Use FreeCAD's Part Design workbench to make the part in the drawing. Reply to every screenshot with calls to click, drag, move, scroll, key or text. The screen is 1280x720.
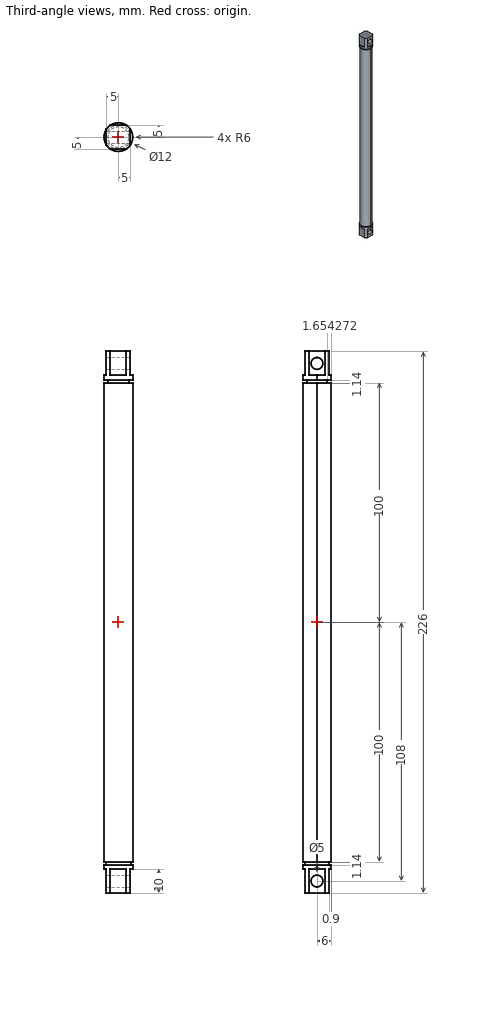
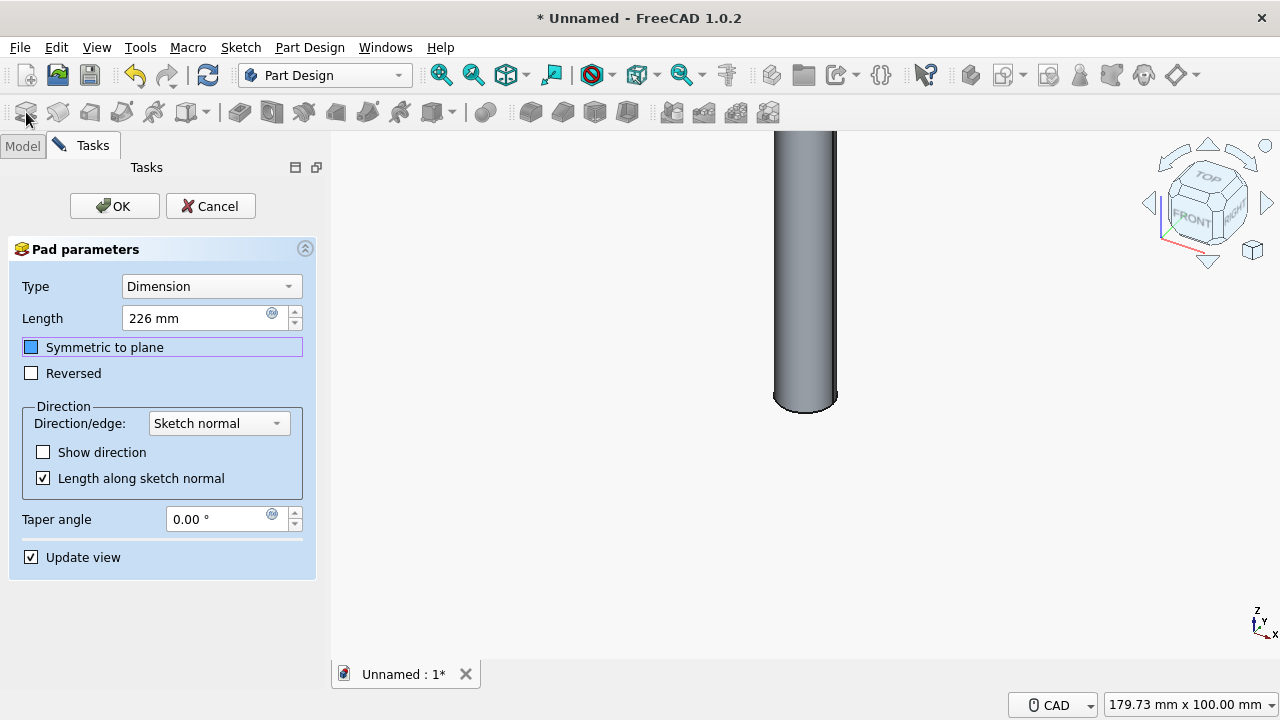
click(30, 347)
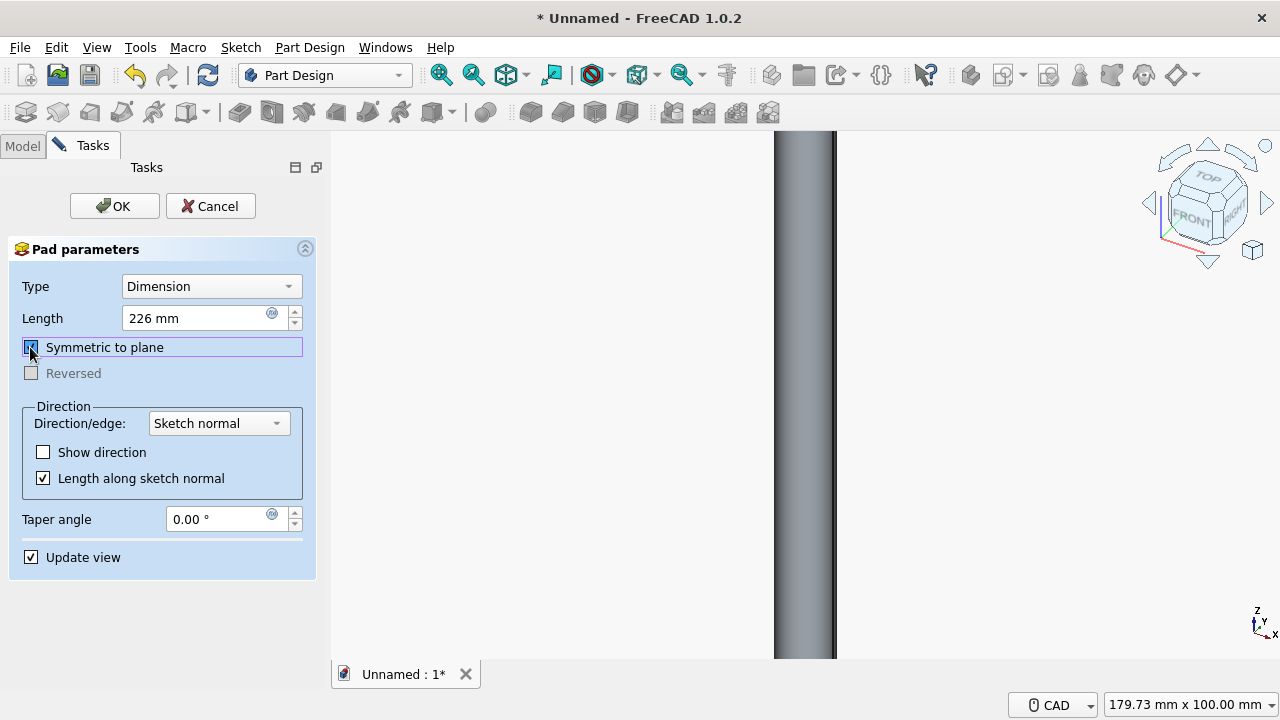
click(115, 206)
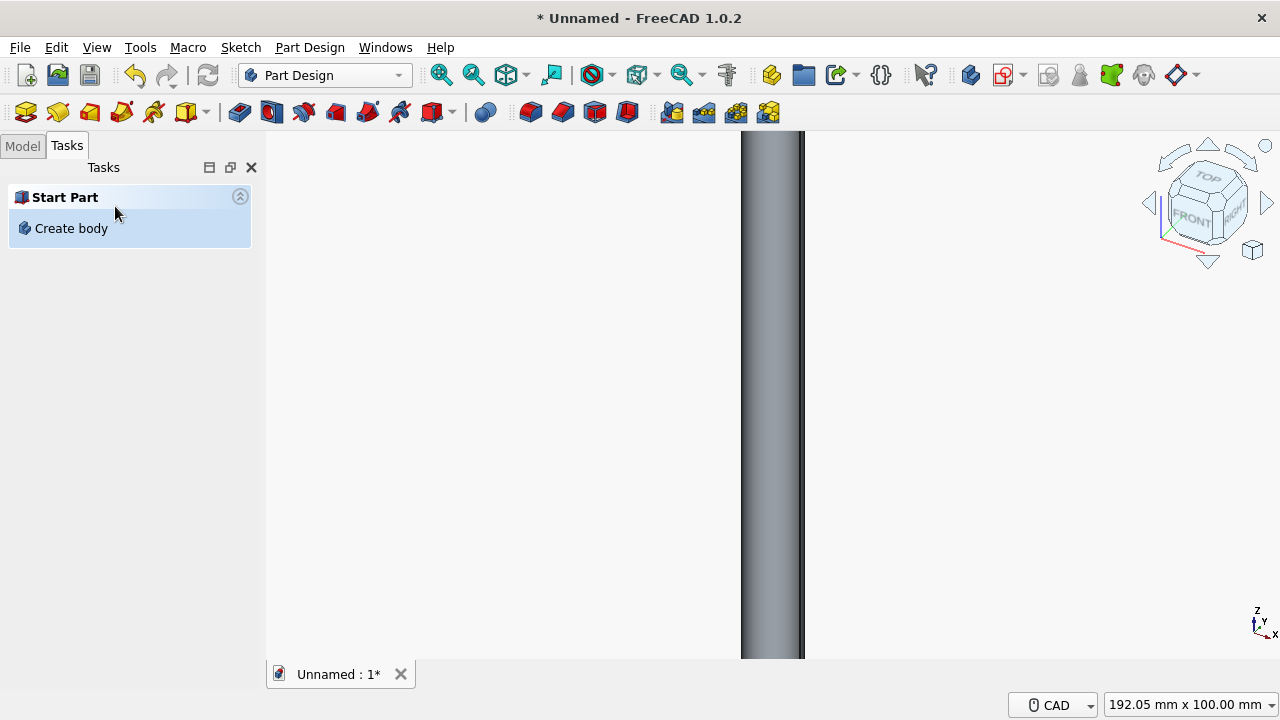
key(v)
key(f)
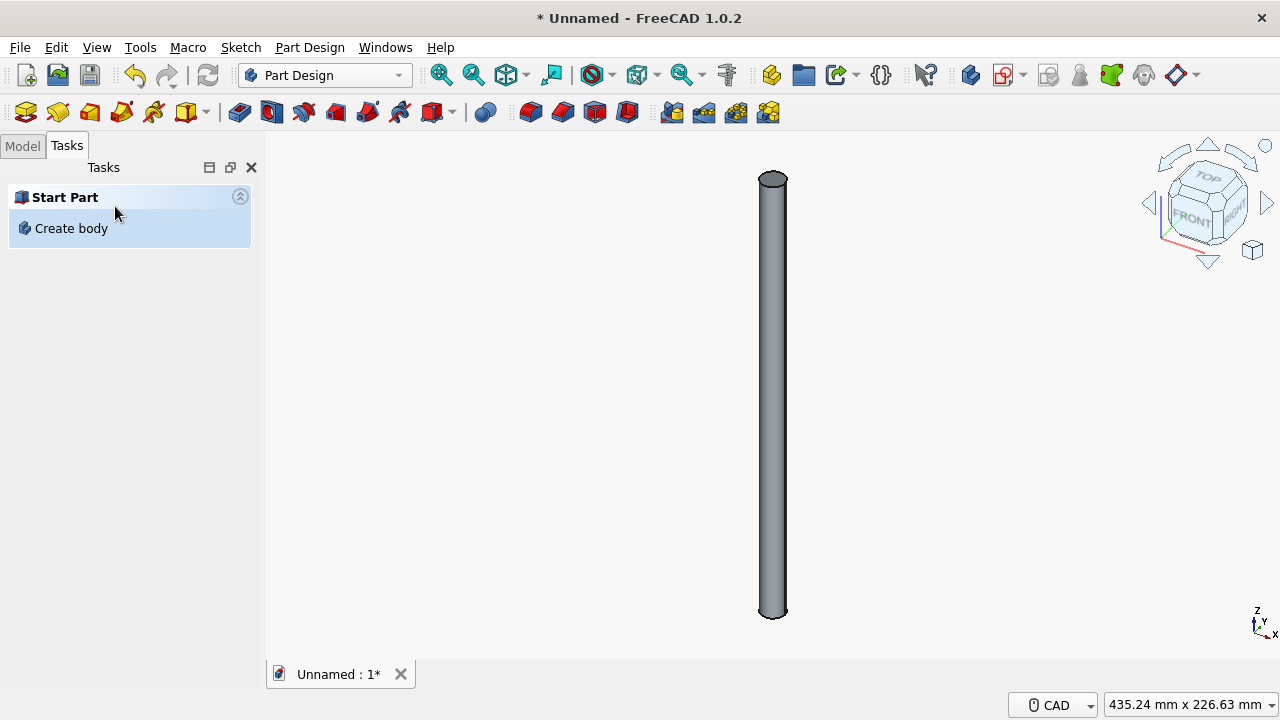
click(1004, 76)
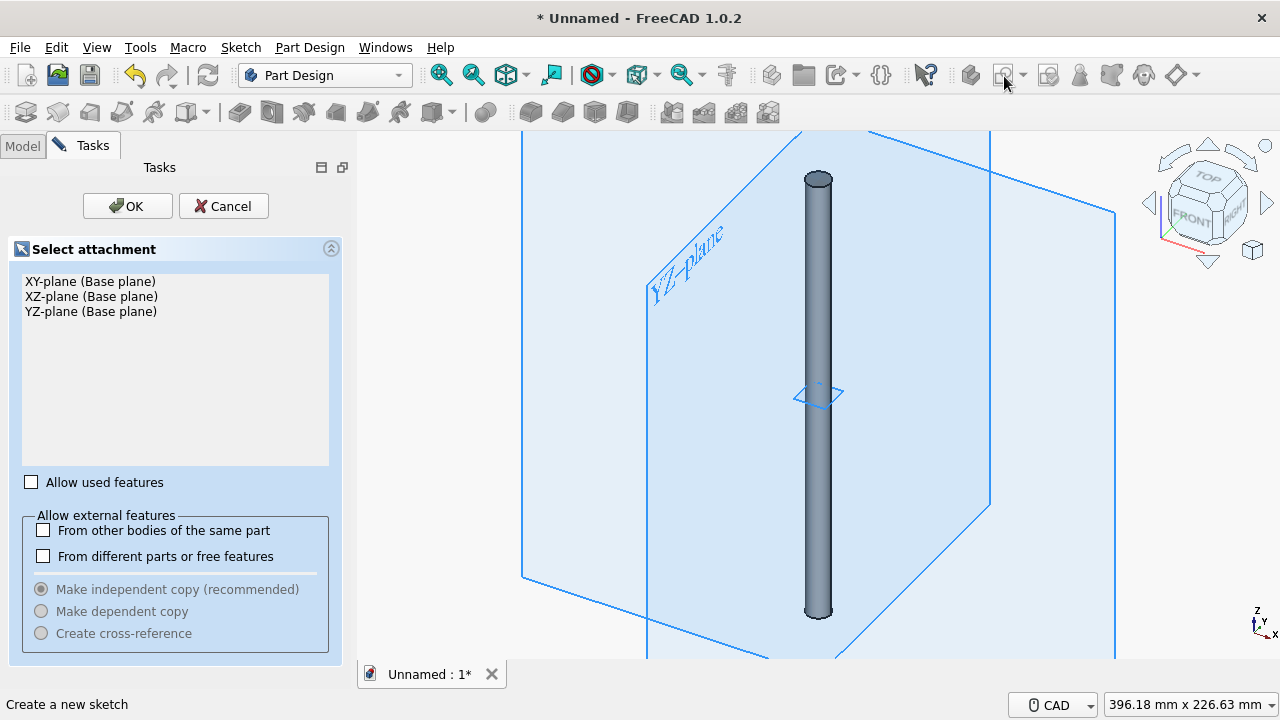
click(82, 312)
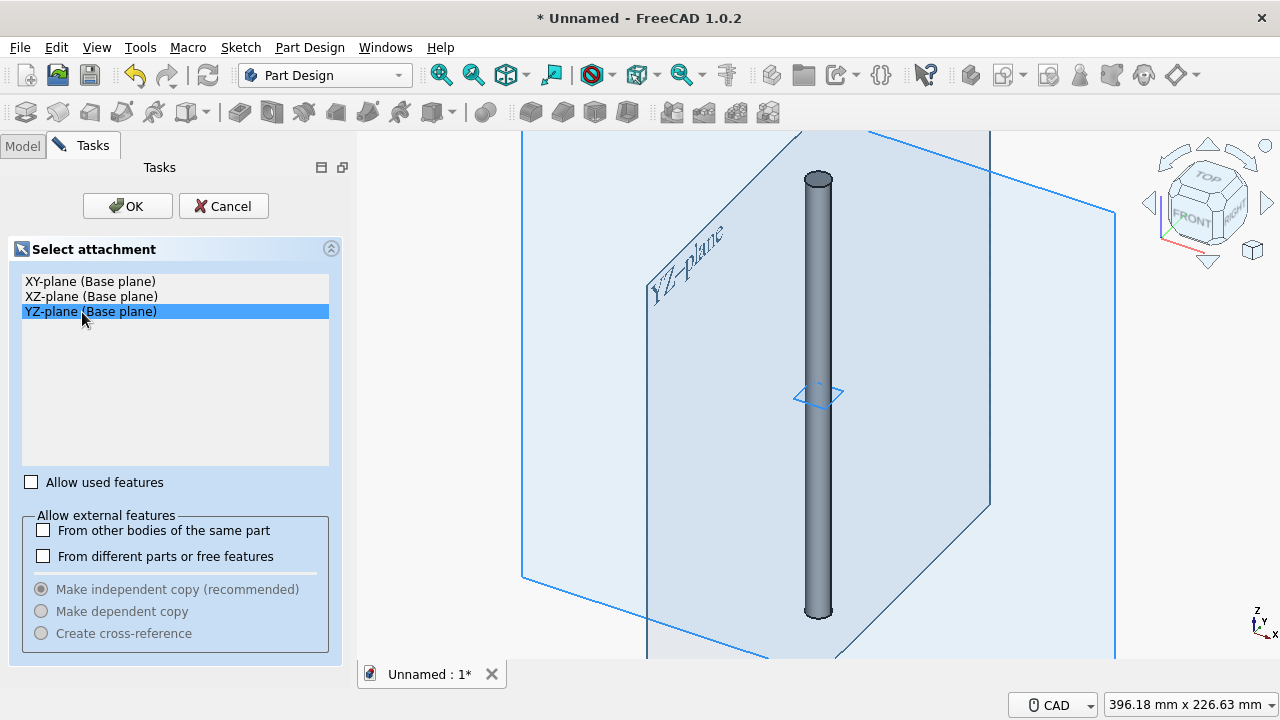
click(128, 206)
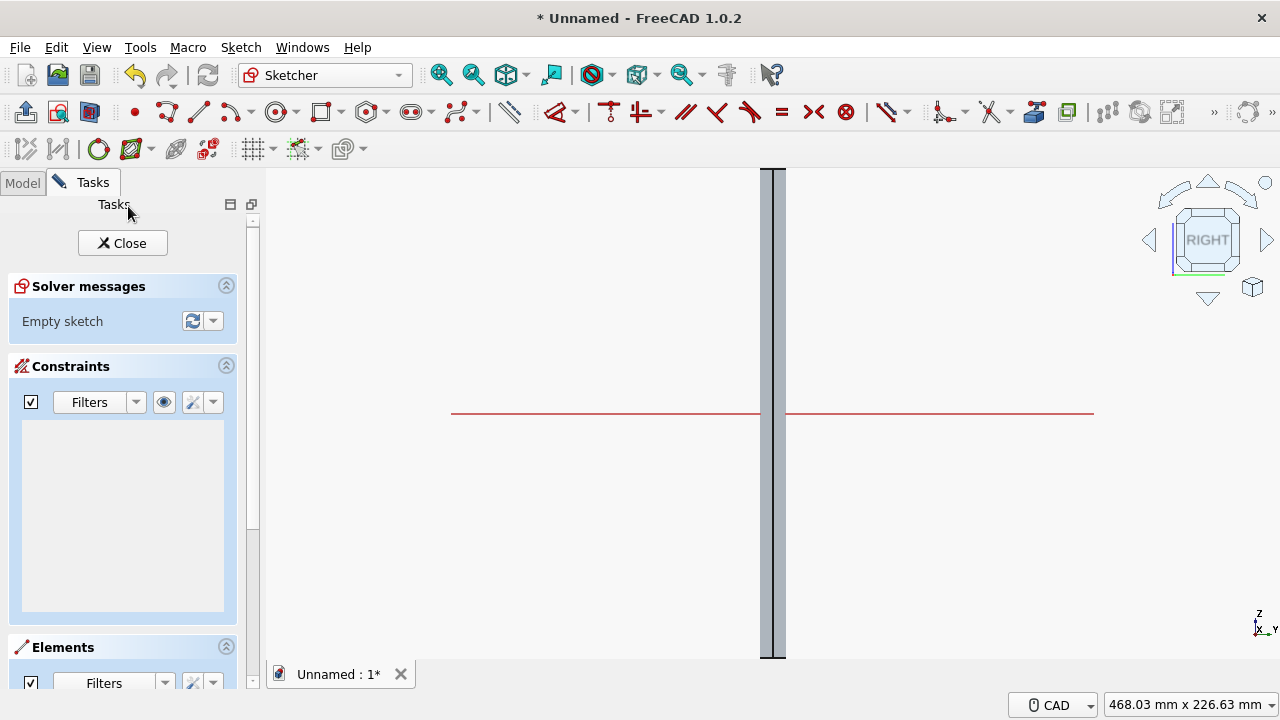
key(q)
key(s)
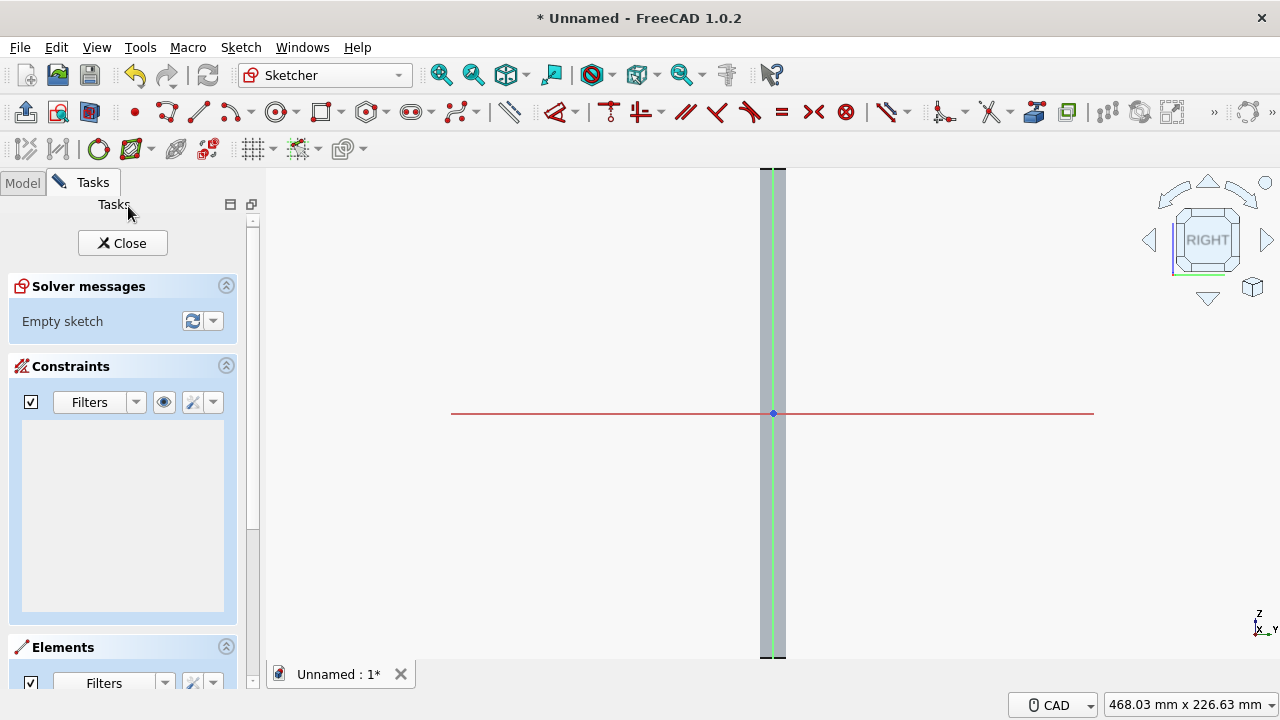
scroll(552, 414, down, 2)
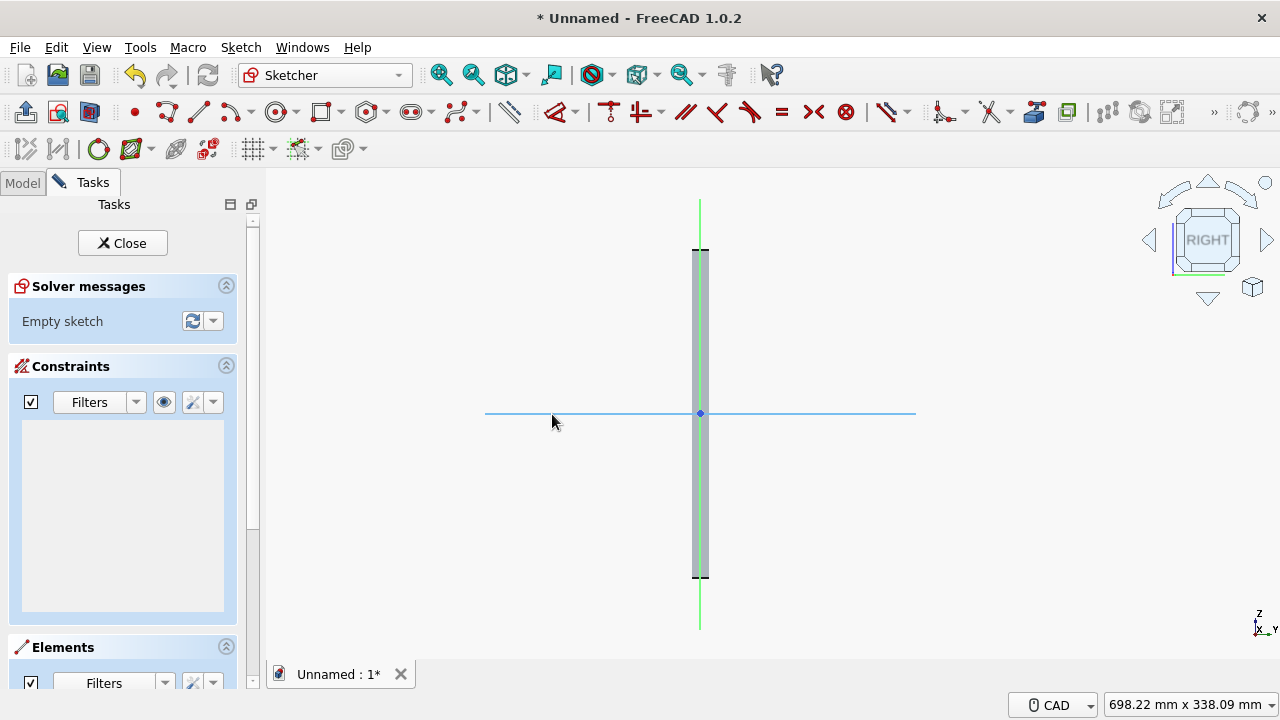
click(322, 112)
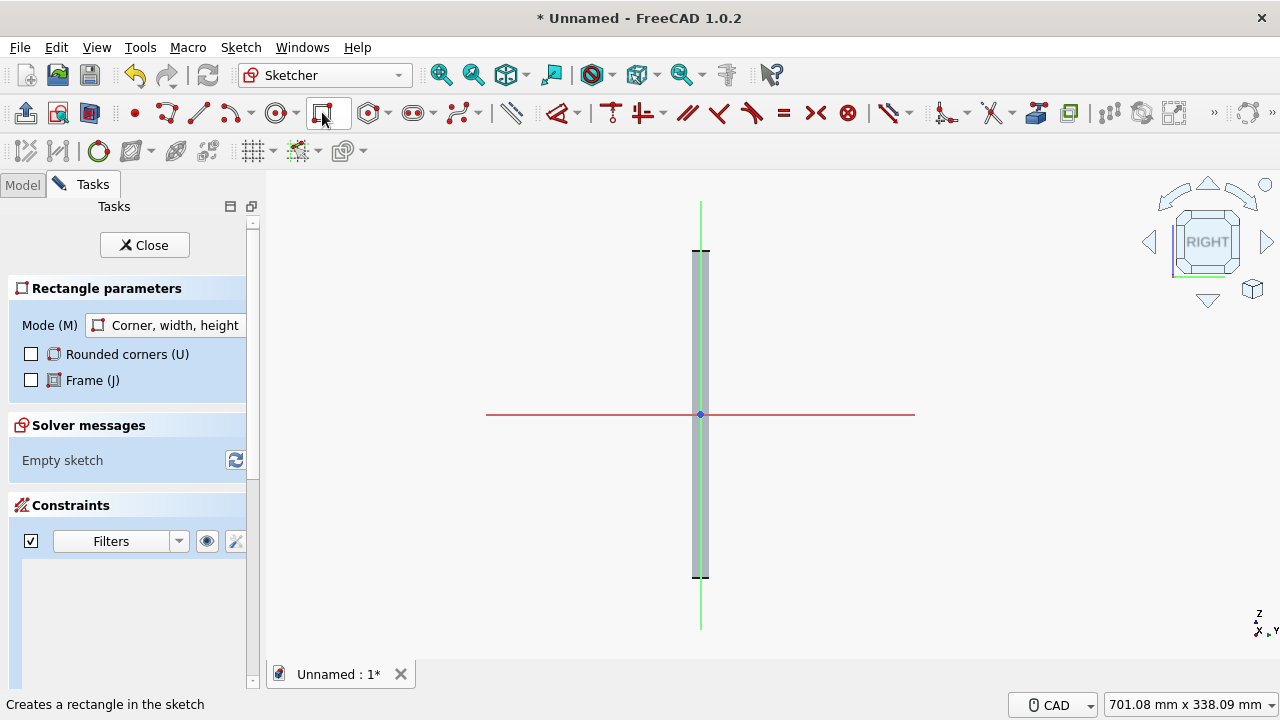
scroll(708, 559, up, 13)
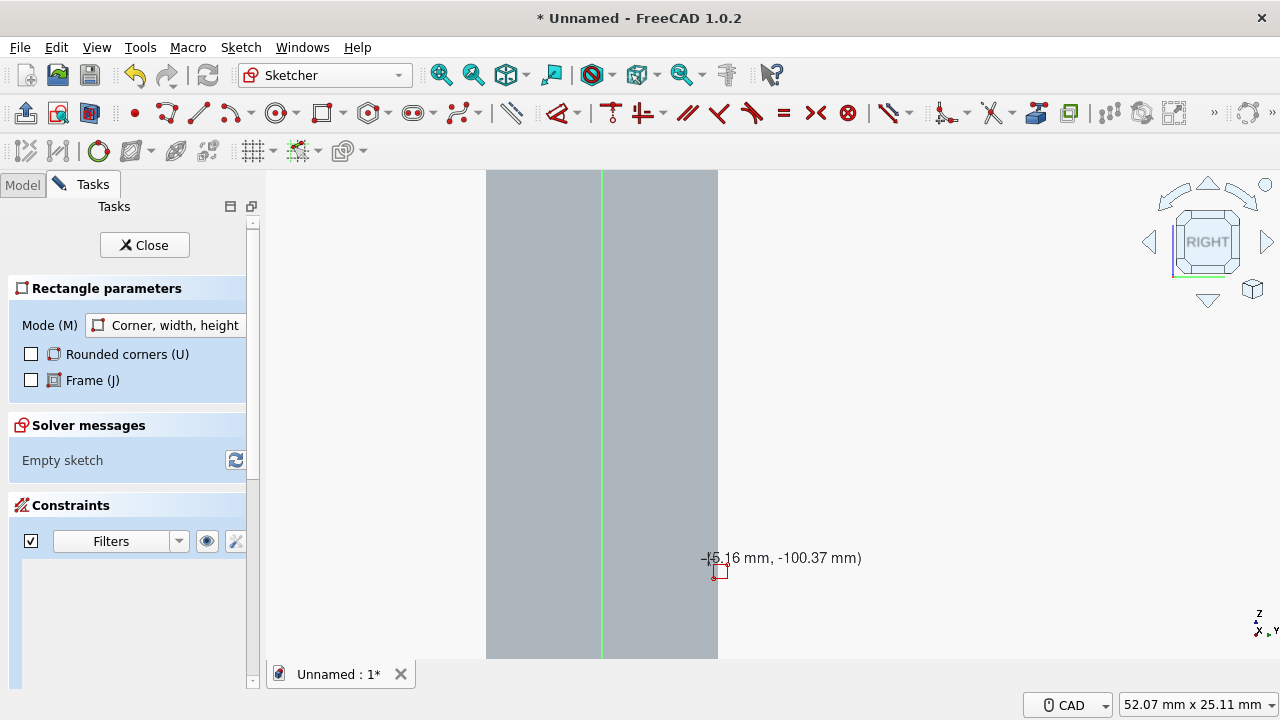
scroll(708, 559, down, 13)